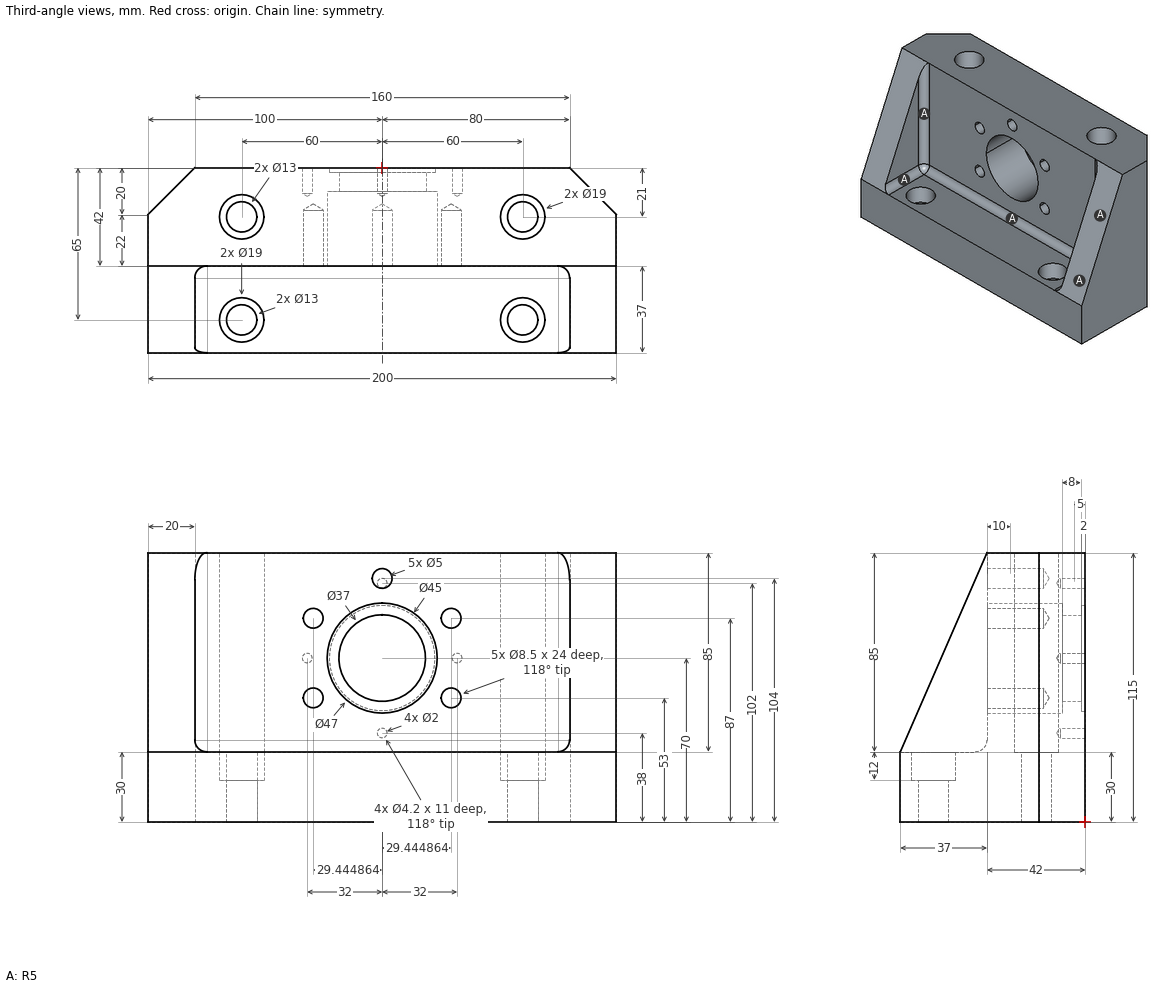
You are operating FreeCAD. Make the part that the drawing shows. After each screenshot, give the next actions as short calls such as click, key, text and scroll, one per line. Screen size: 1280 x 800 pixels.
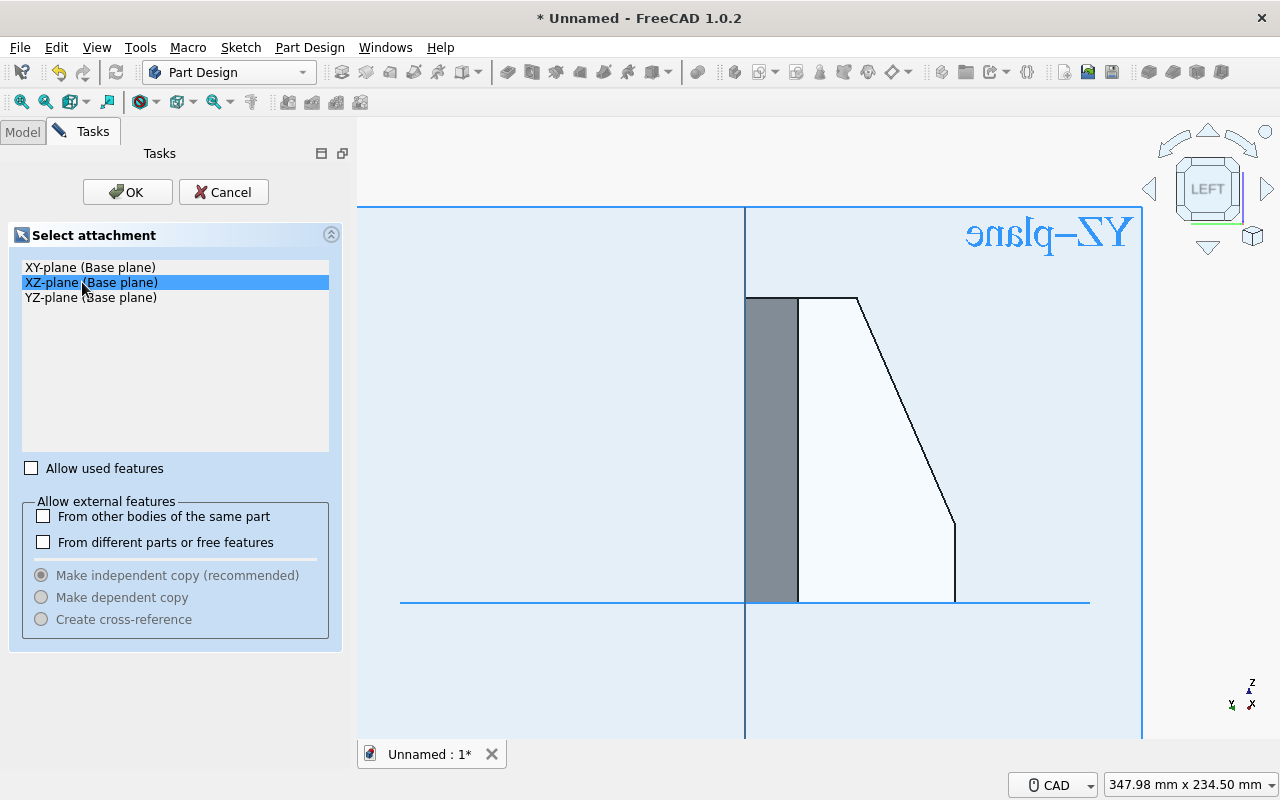
click(128, 192)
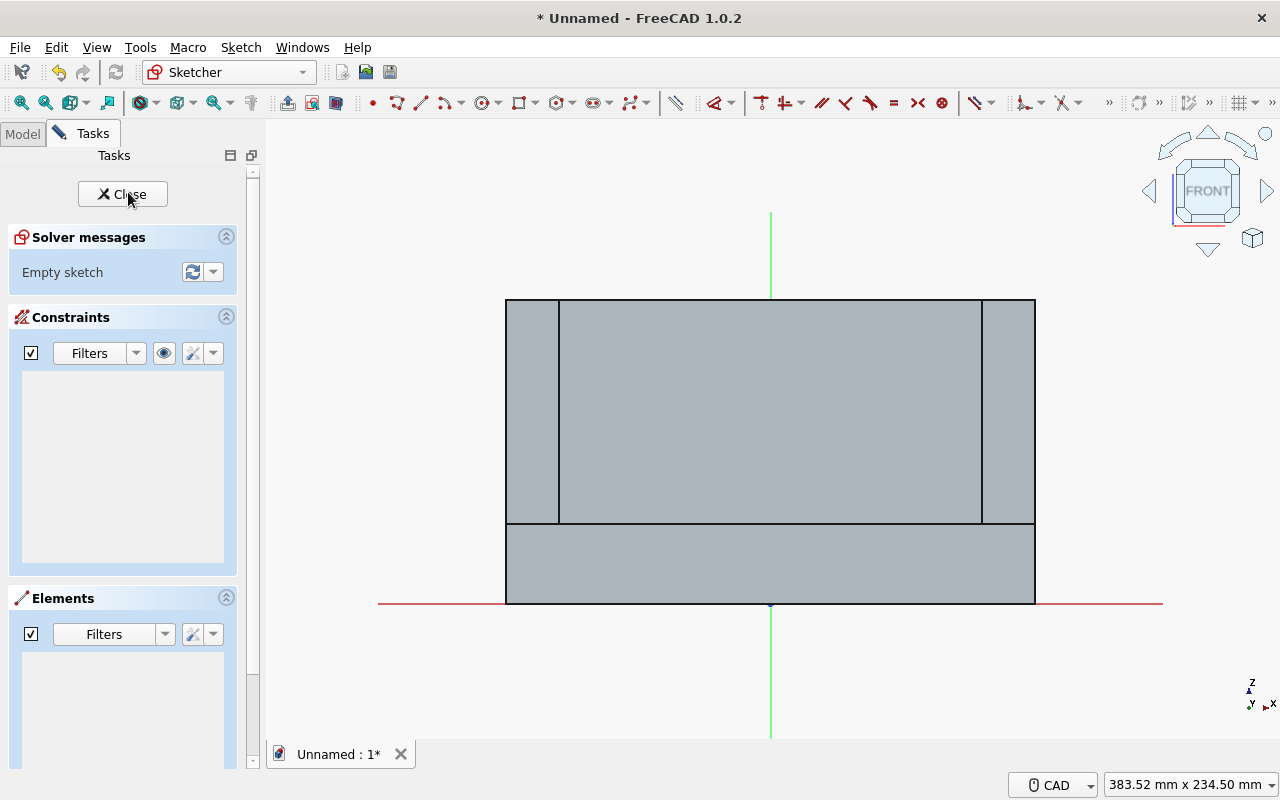
click(336, 104)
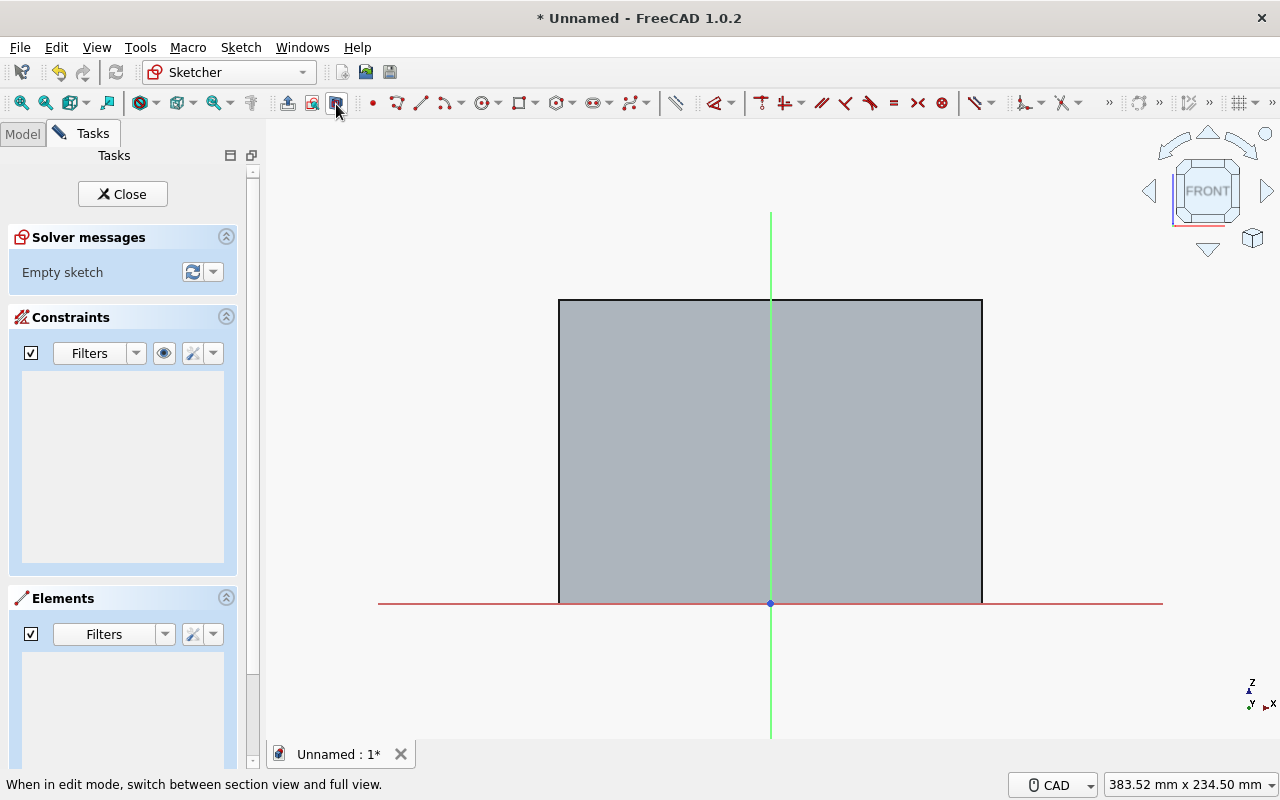
scroll(905, 588, up, 2)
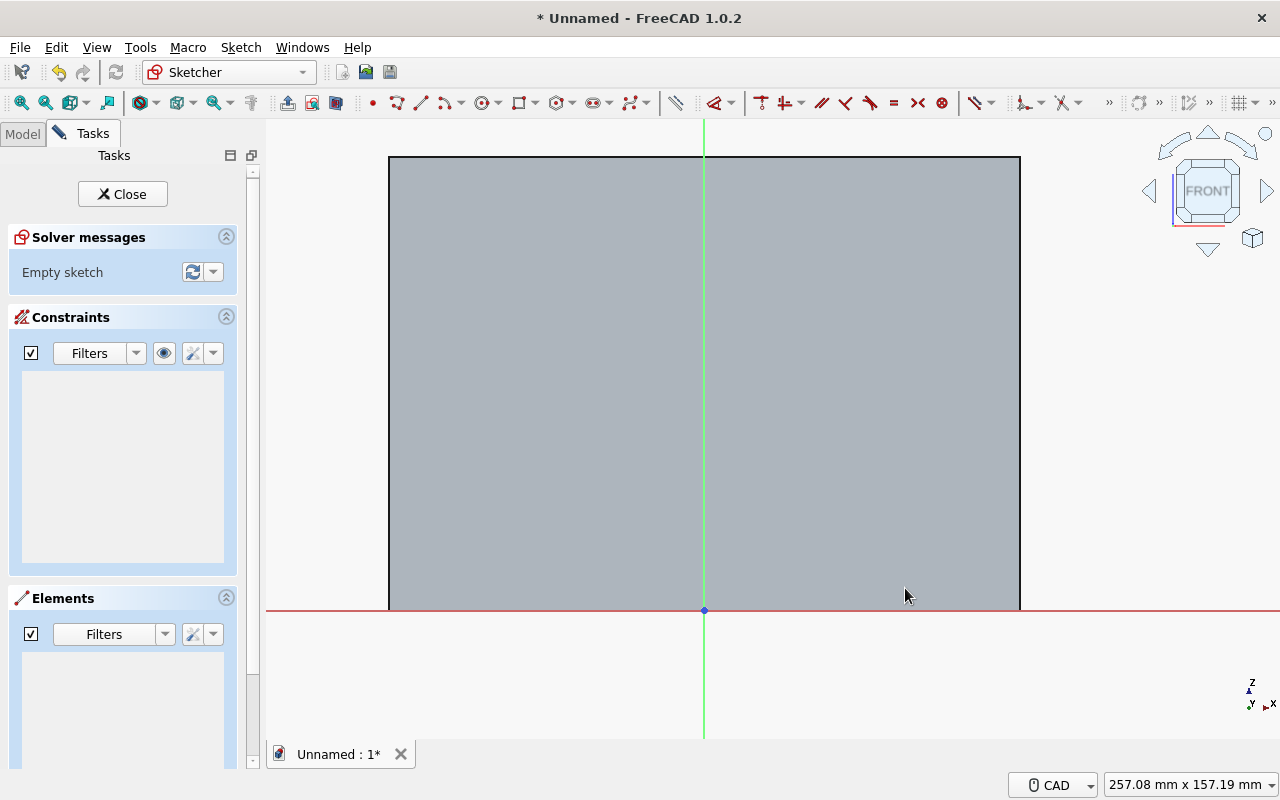
click(482, 104)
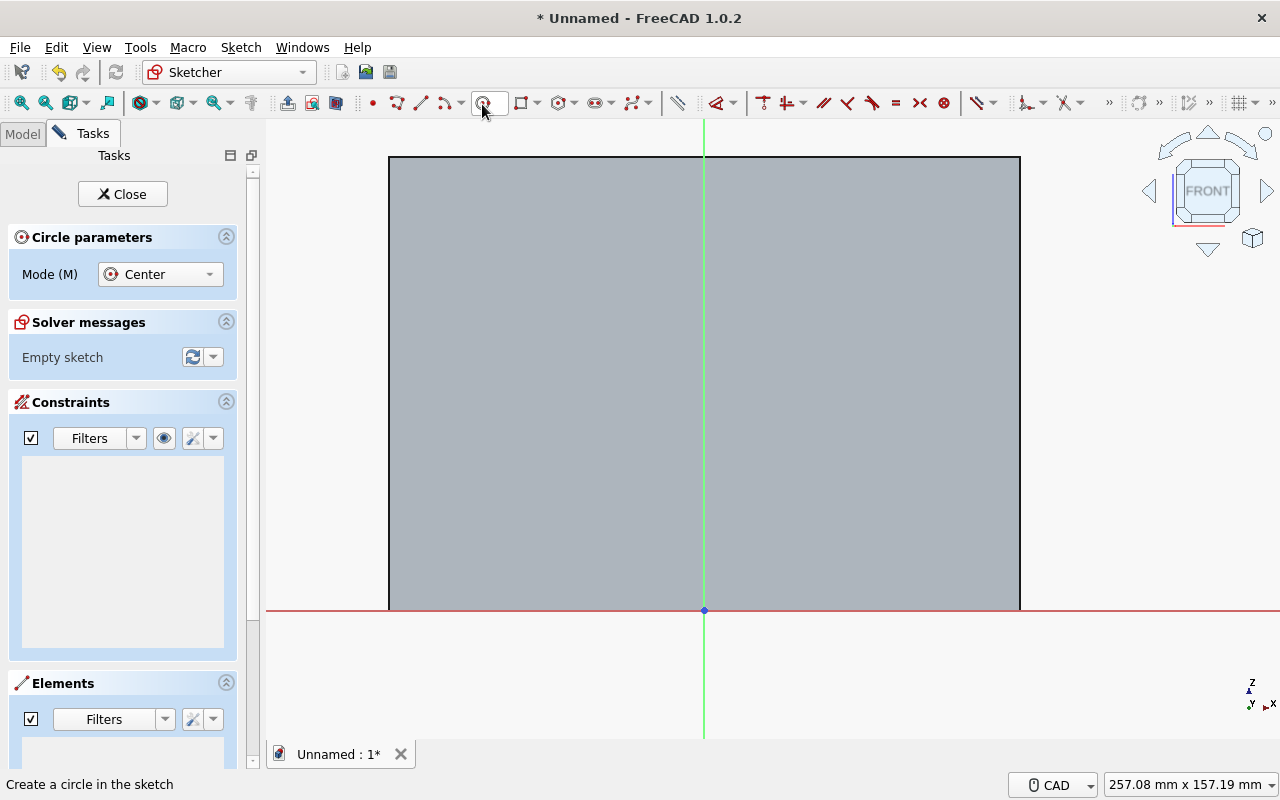
click(704, 335)
move(767, 272)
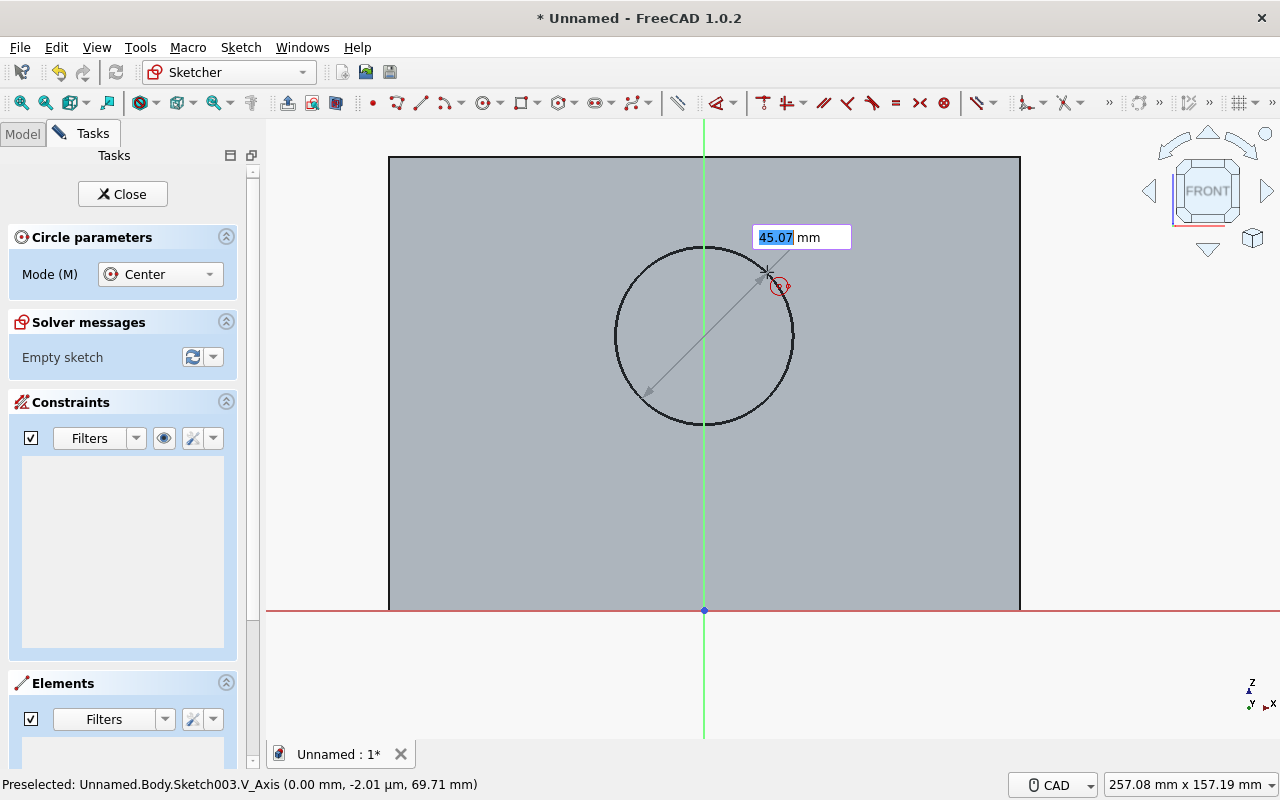
text(45)
key(Return)
key(Escape)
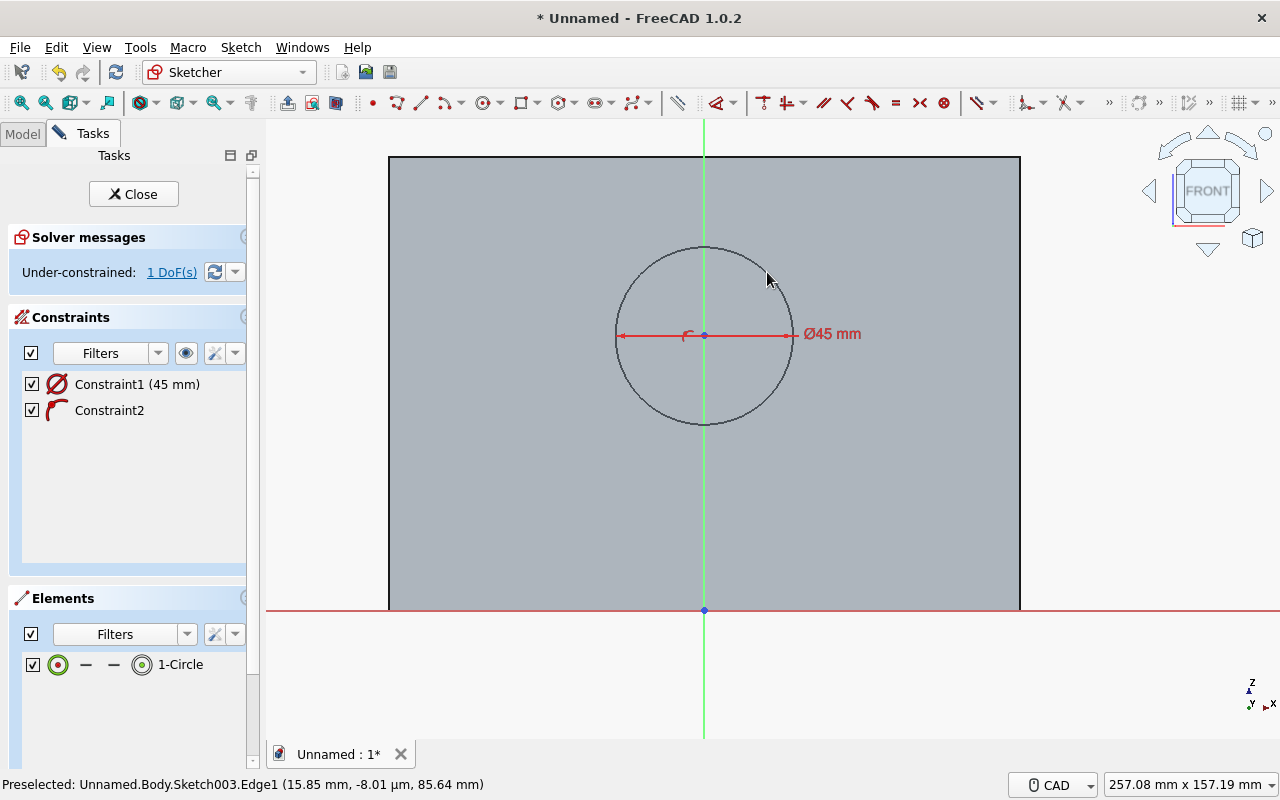
click(716, 104)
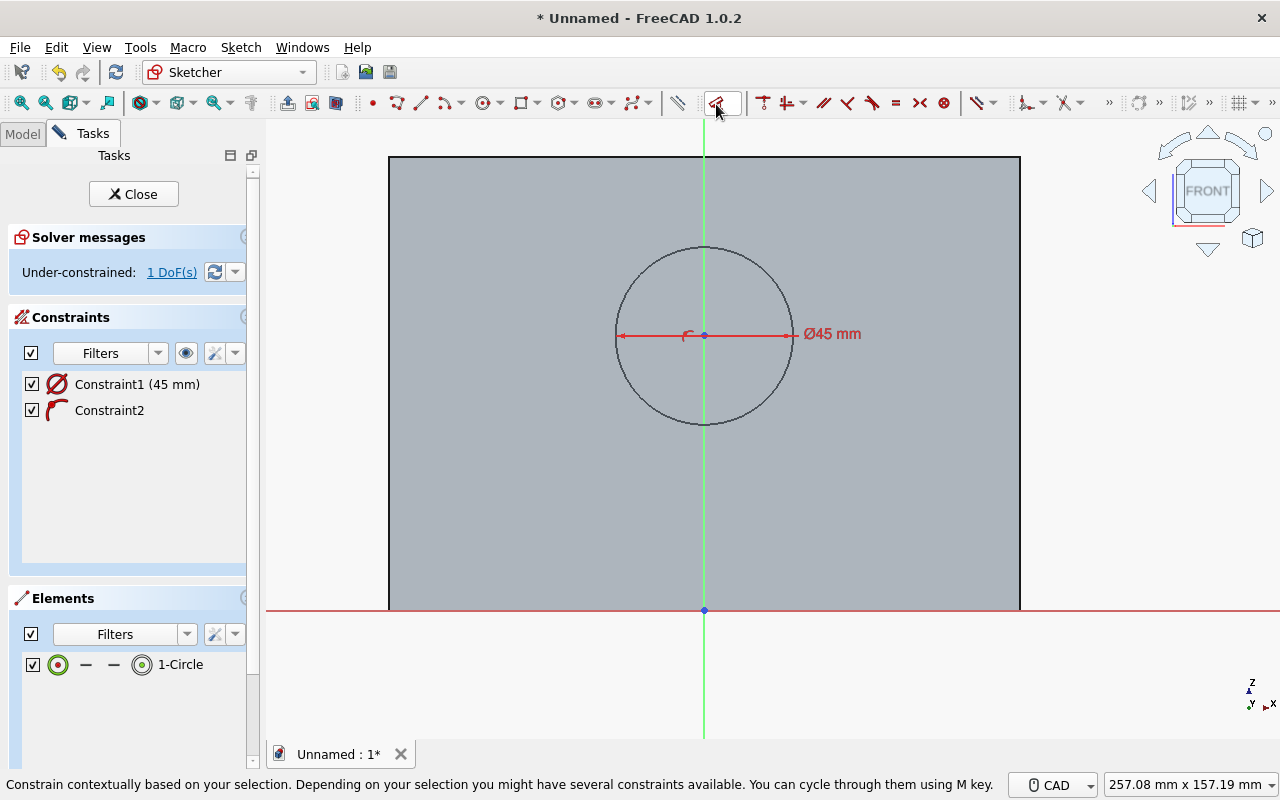
click(704, 336)
click(738, 473)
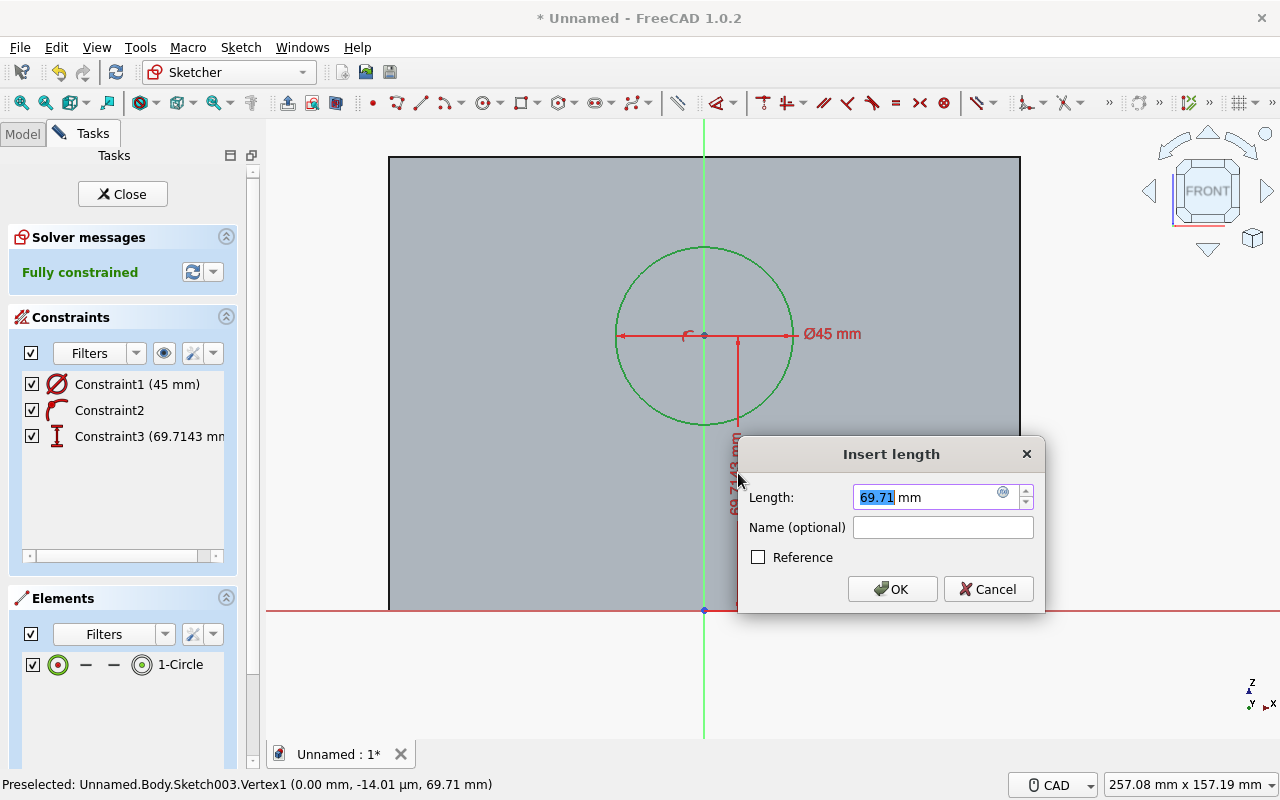
text(70)
key(Return)
key(Escape)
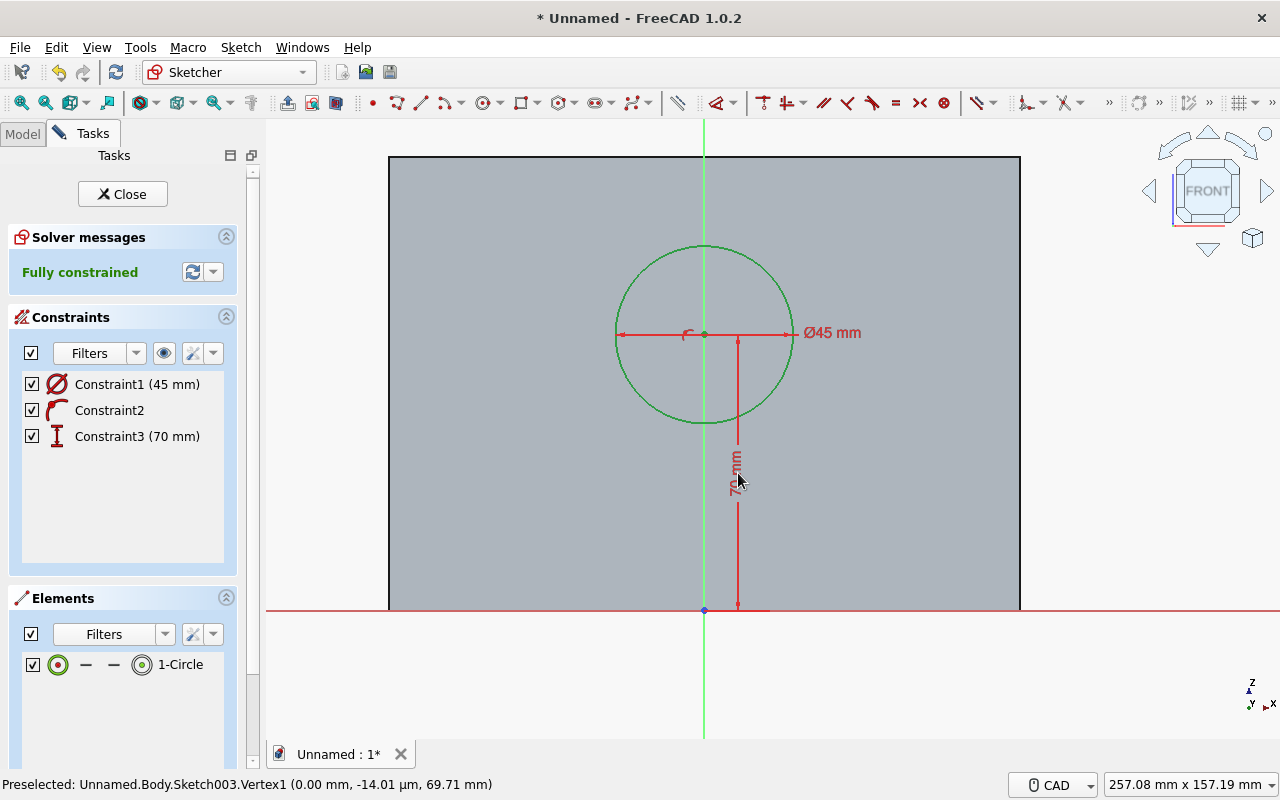
click(123, 194)